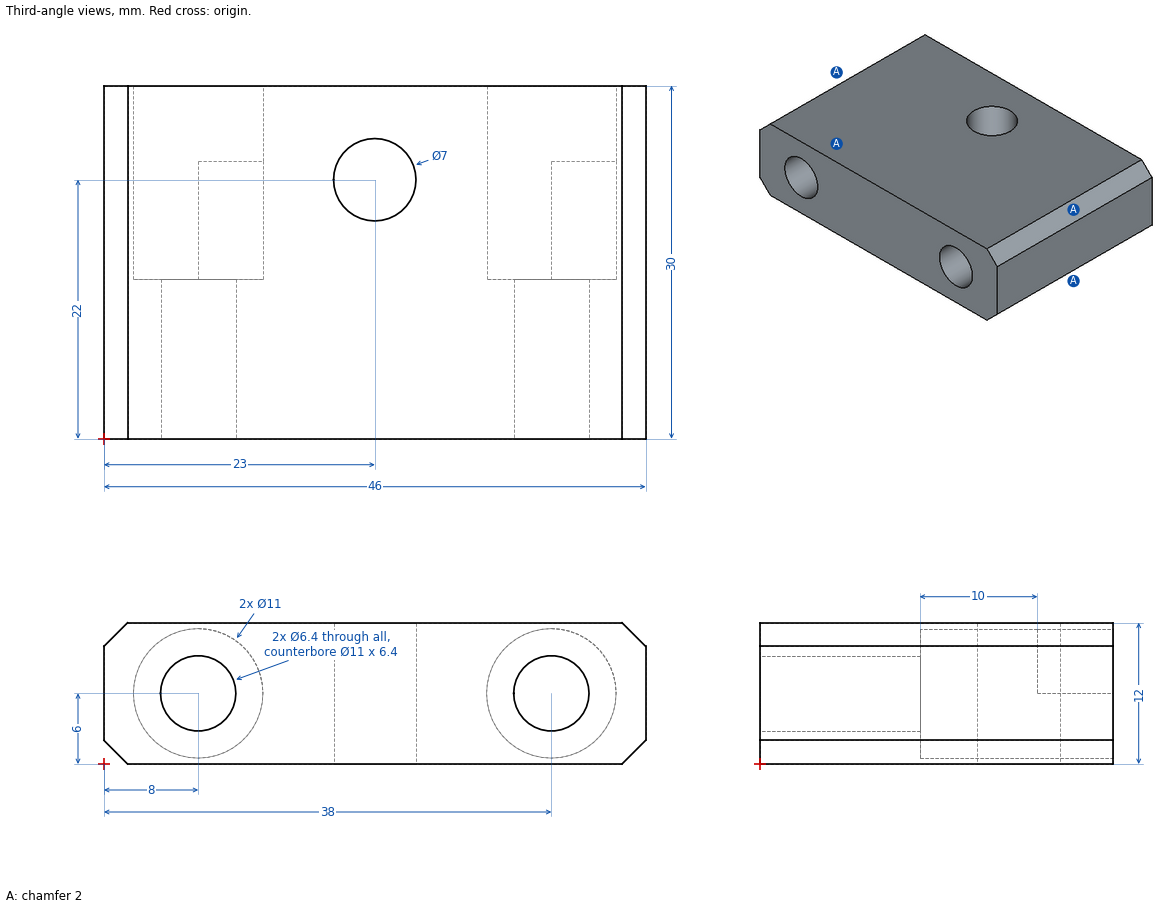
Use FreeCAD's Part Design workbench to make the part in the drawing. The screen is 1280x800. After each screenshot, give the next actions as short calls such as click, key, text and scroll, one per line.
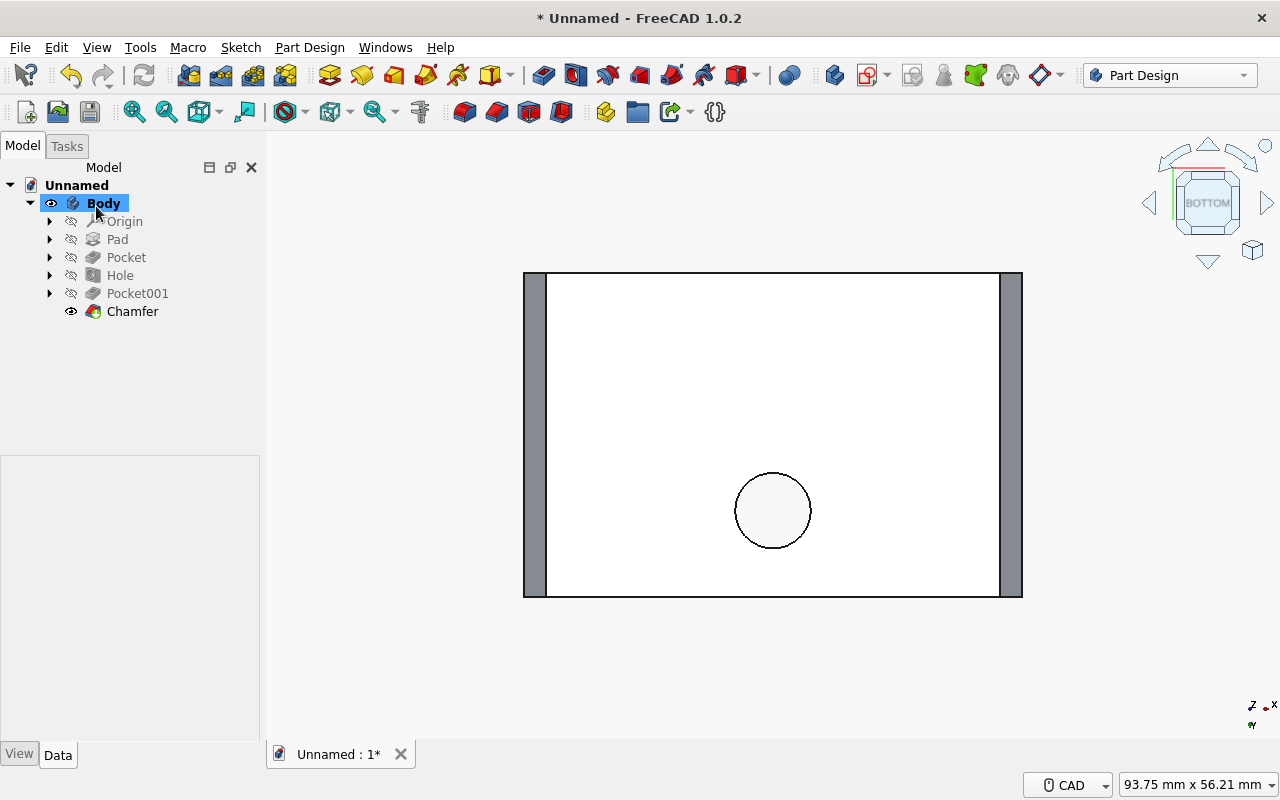
key(0)